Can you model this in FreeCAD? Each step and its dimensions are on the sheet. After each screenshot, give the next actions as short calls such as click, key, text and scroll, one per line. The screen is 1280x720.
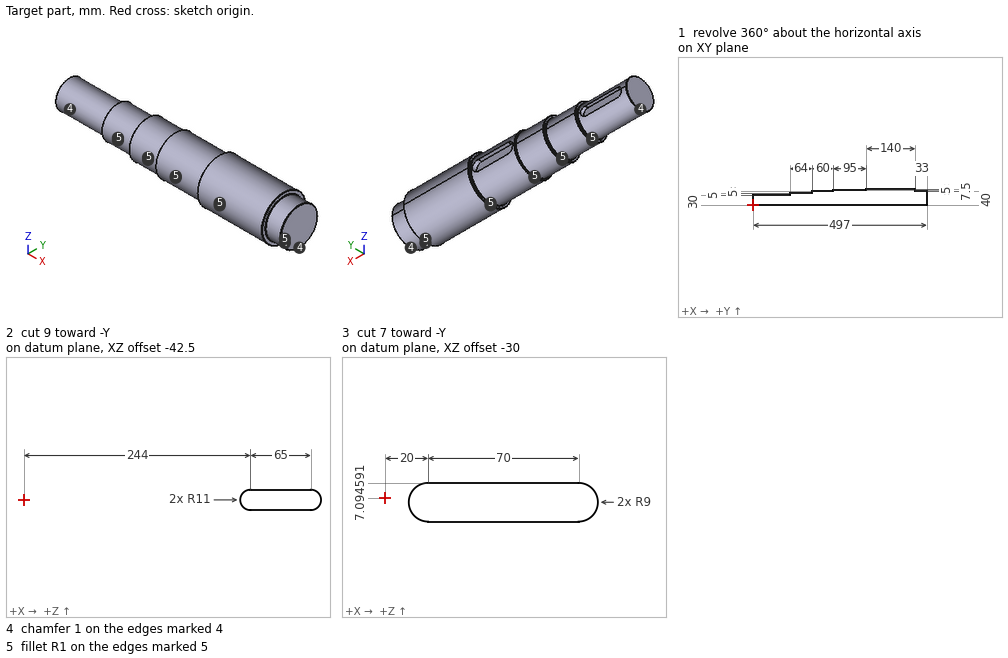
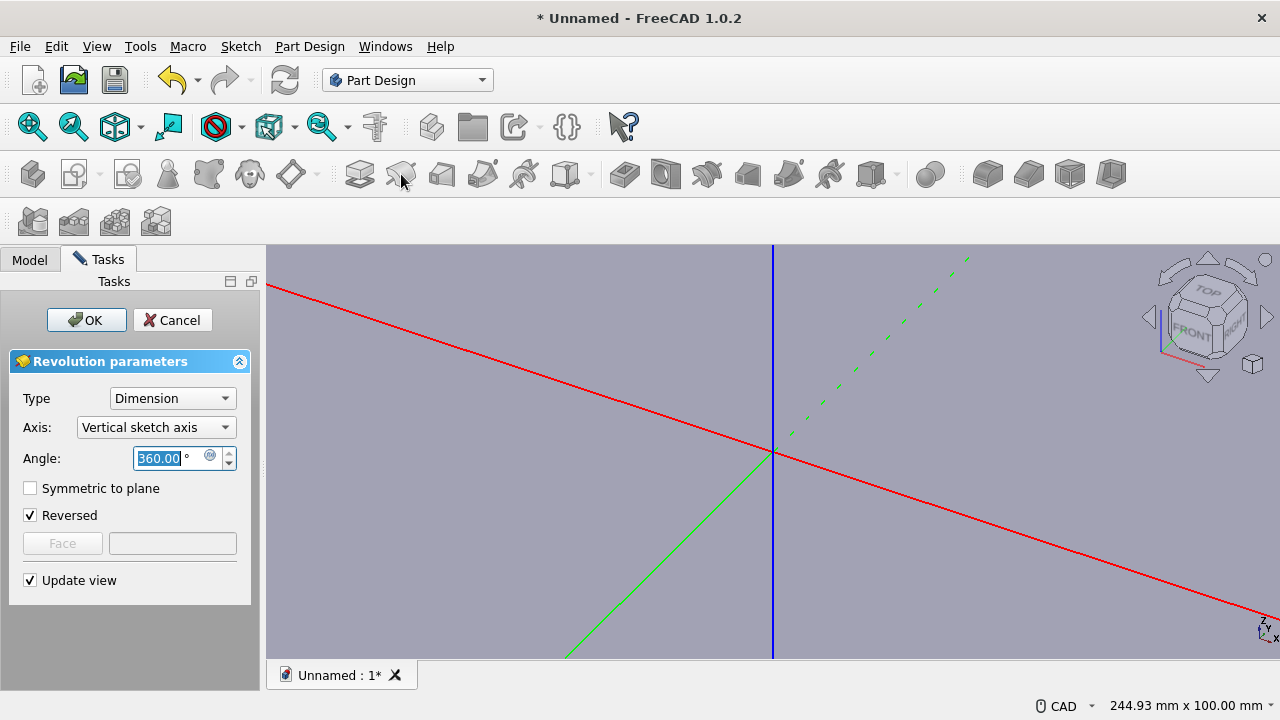
click(157, 428)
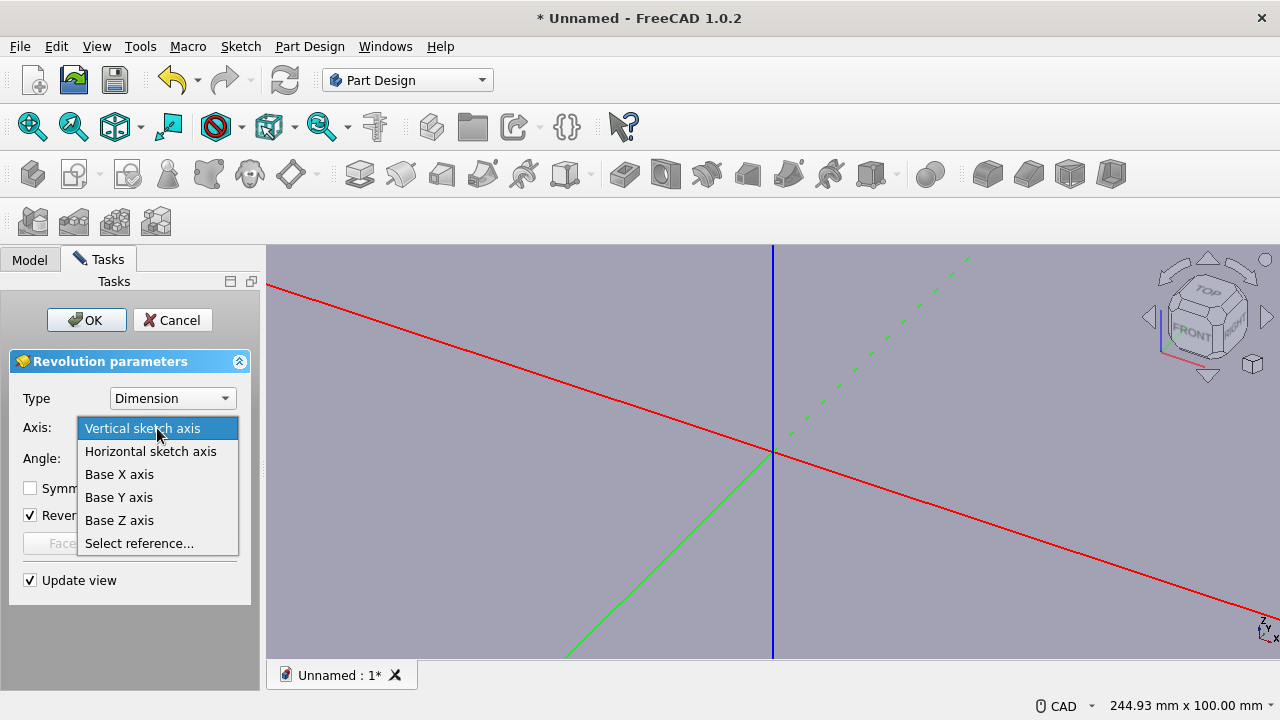
click(156, 452)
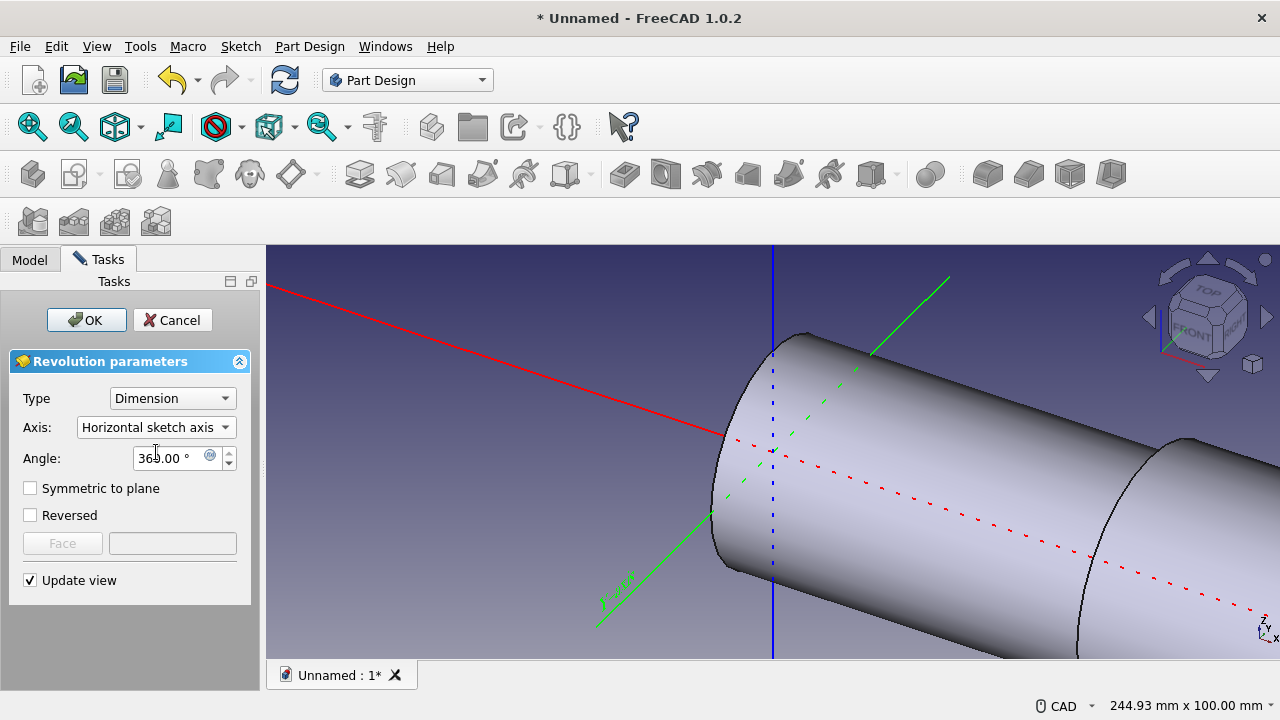
click(87, 320)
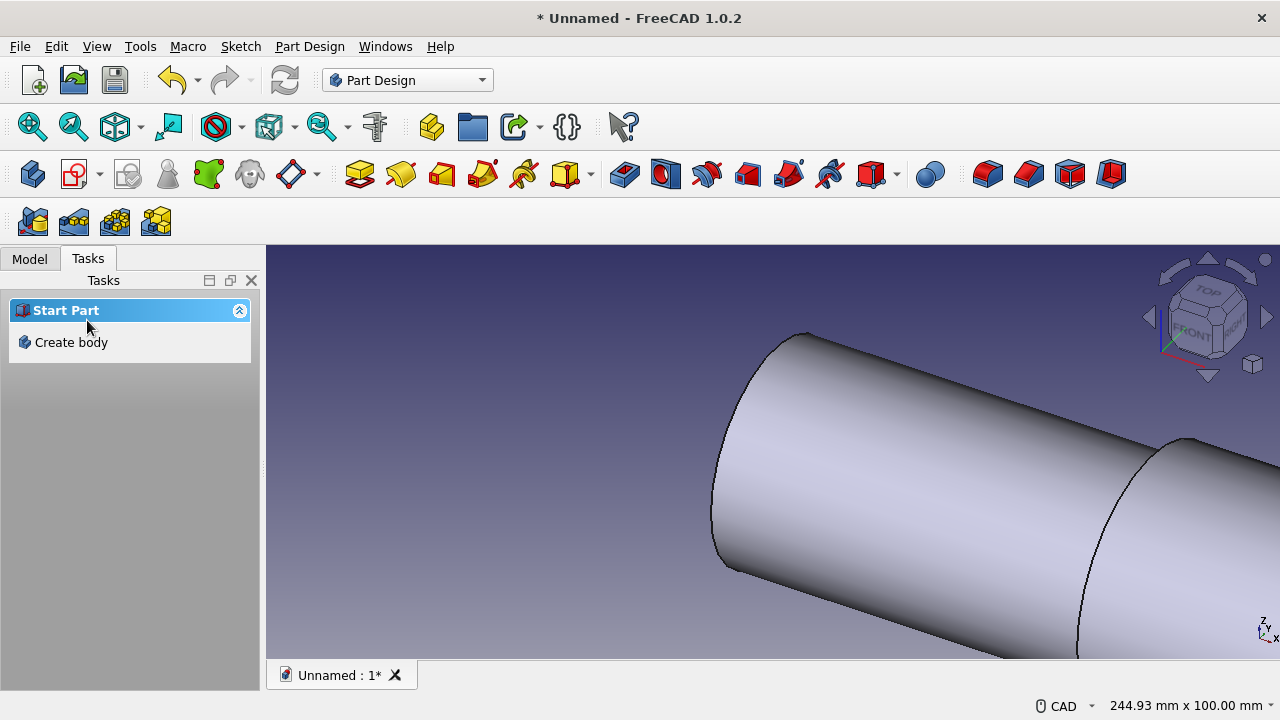
click(33, 128)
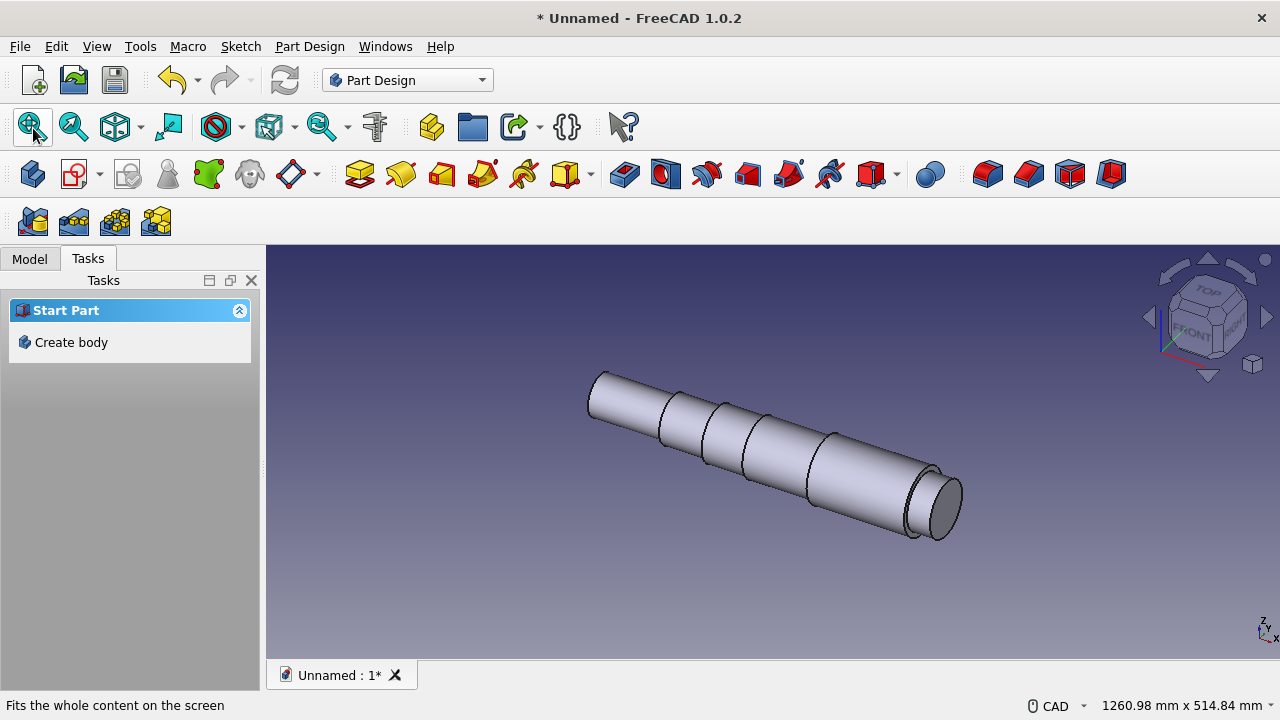
click(30, 258)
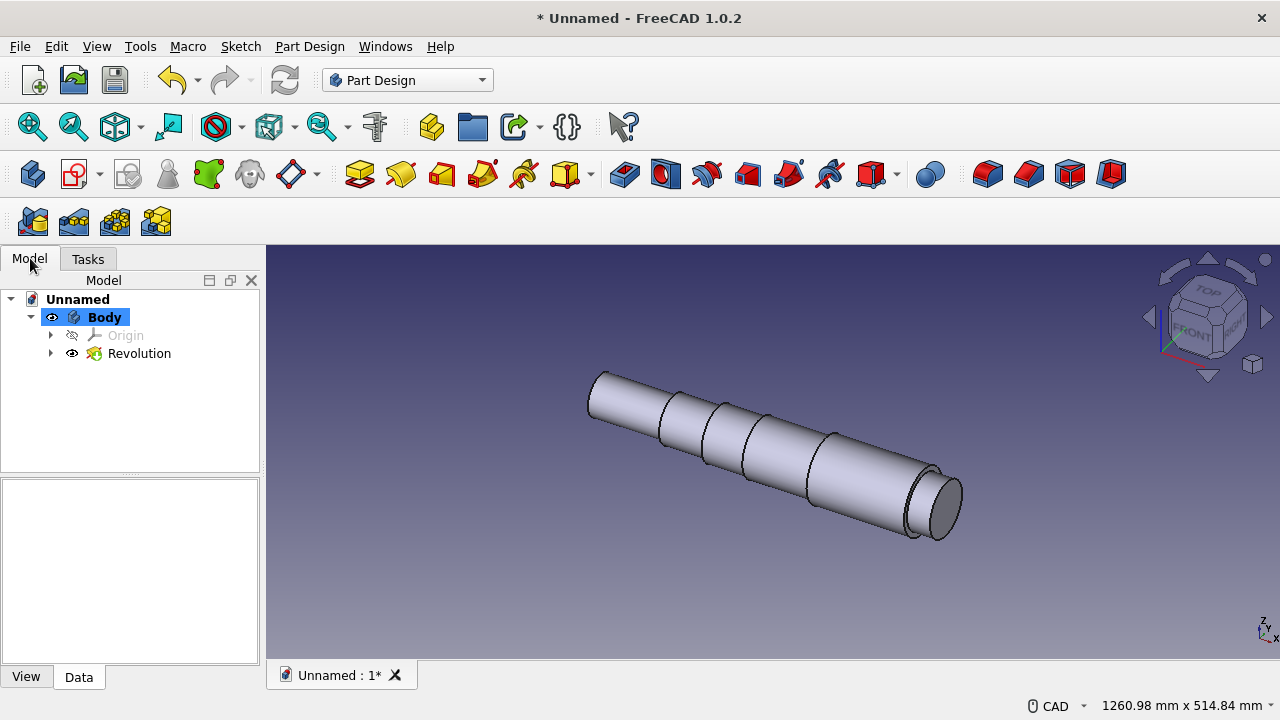
click(51, 335)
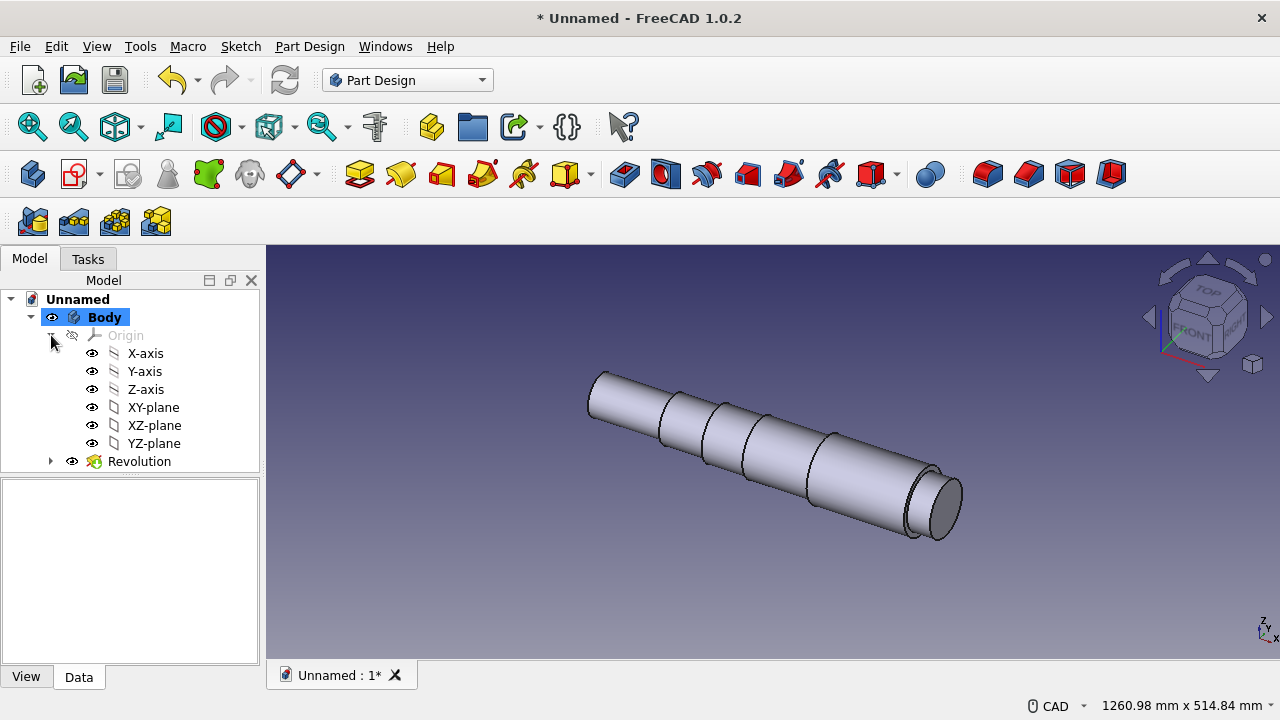
click(137, 425)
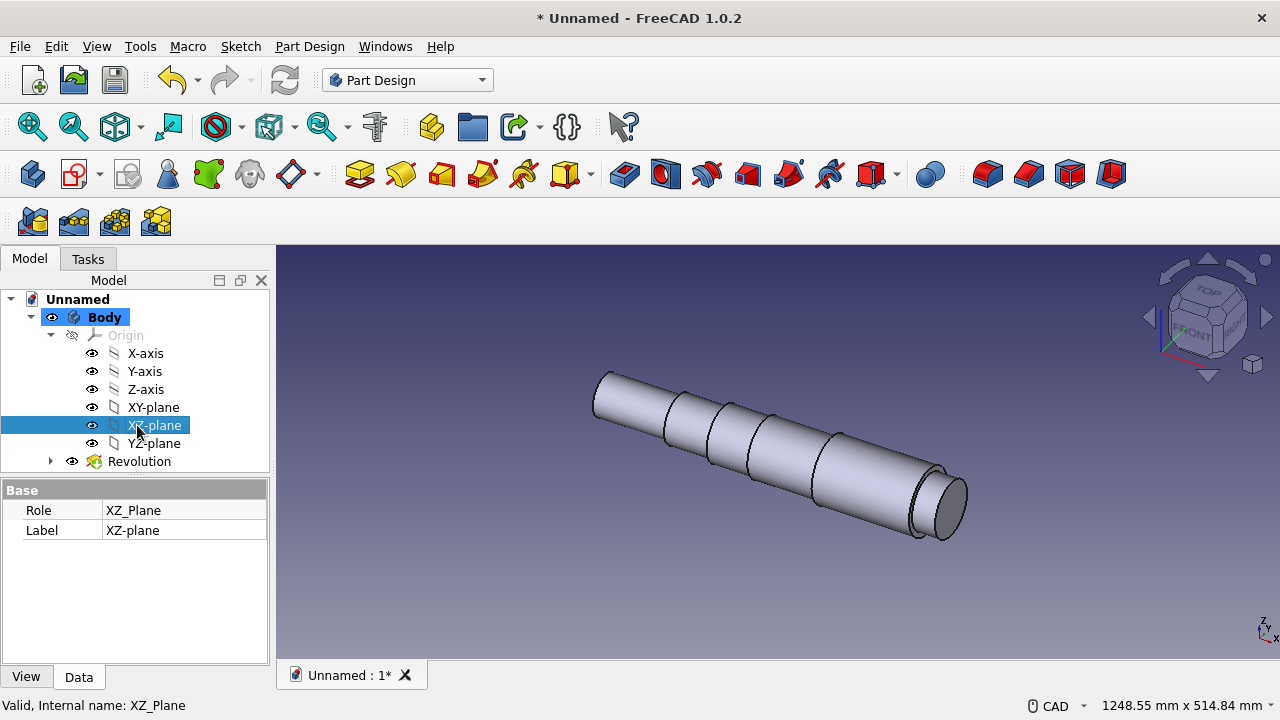
click(290, 174)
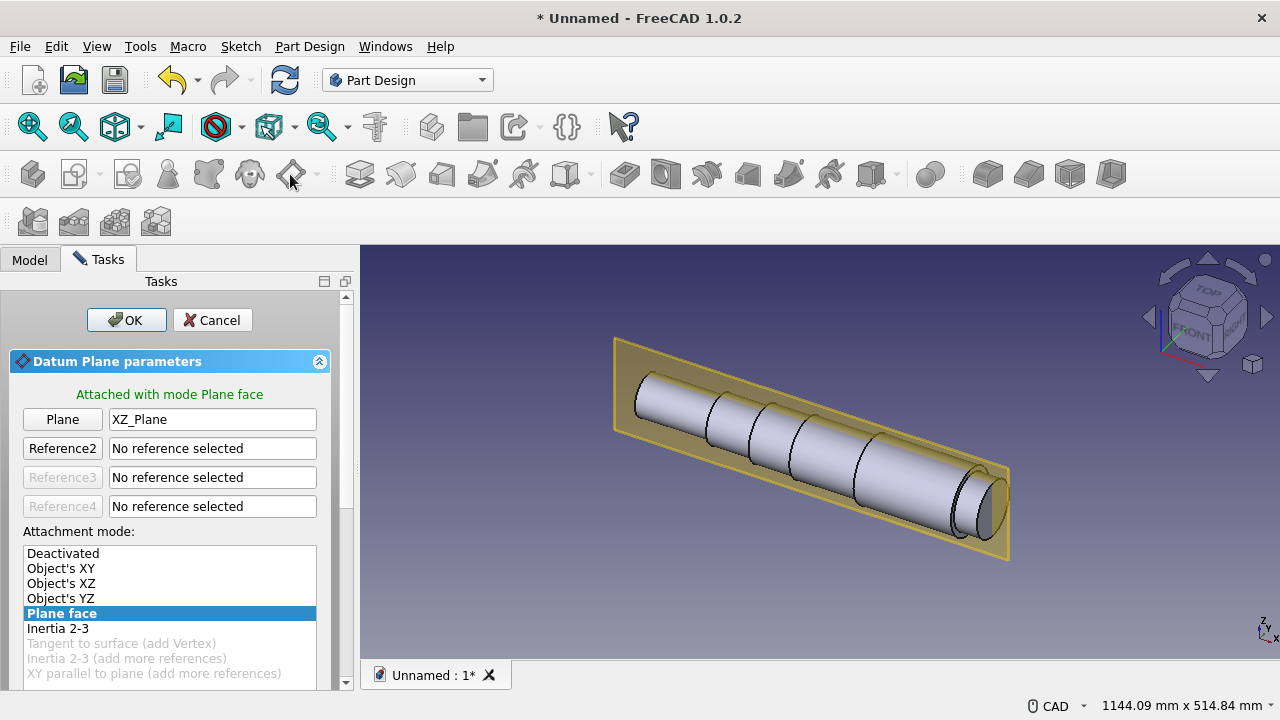
scroll(346, 490, down, 4)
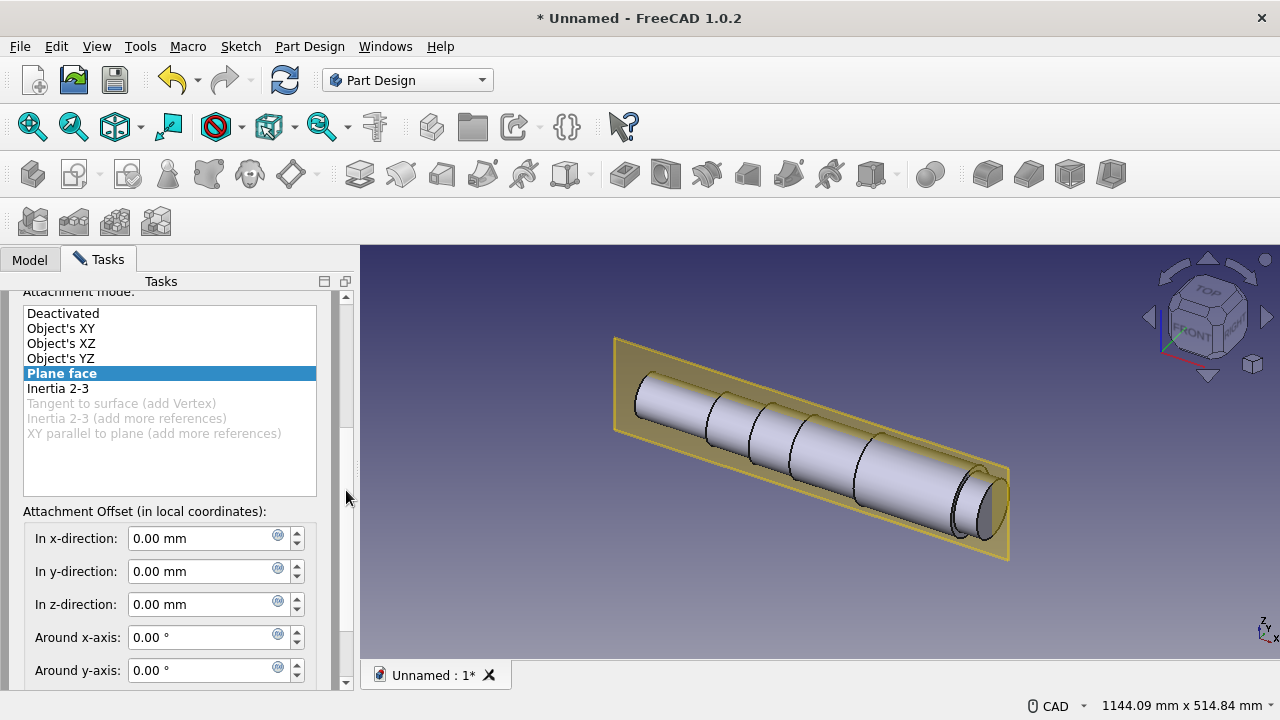
triple_click(210, 604)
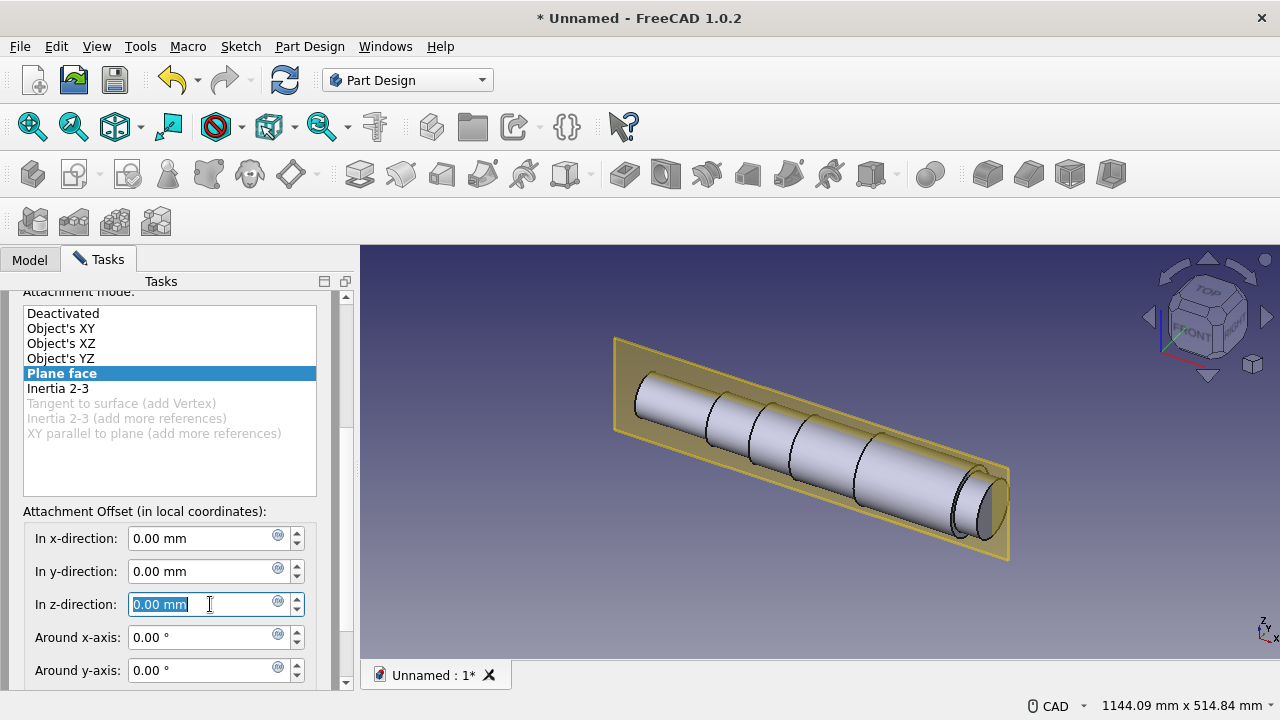
text(-42.5)
key(Tab)